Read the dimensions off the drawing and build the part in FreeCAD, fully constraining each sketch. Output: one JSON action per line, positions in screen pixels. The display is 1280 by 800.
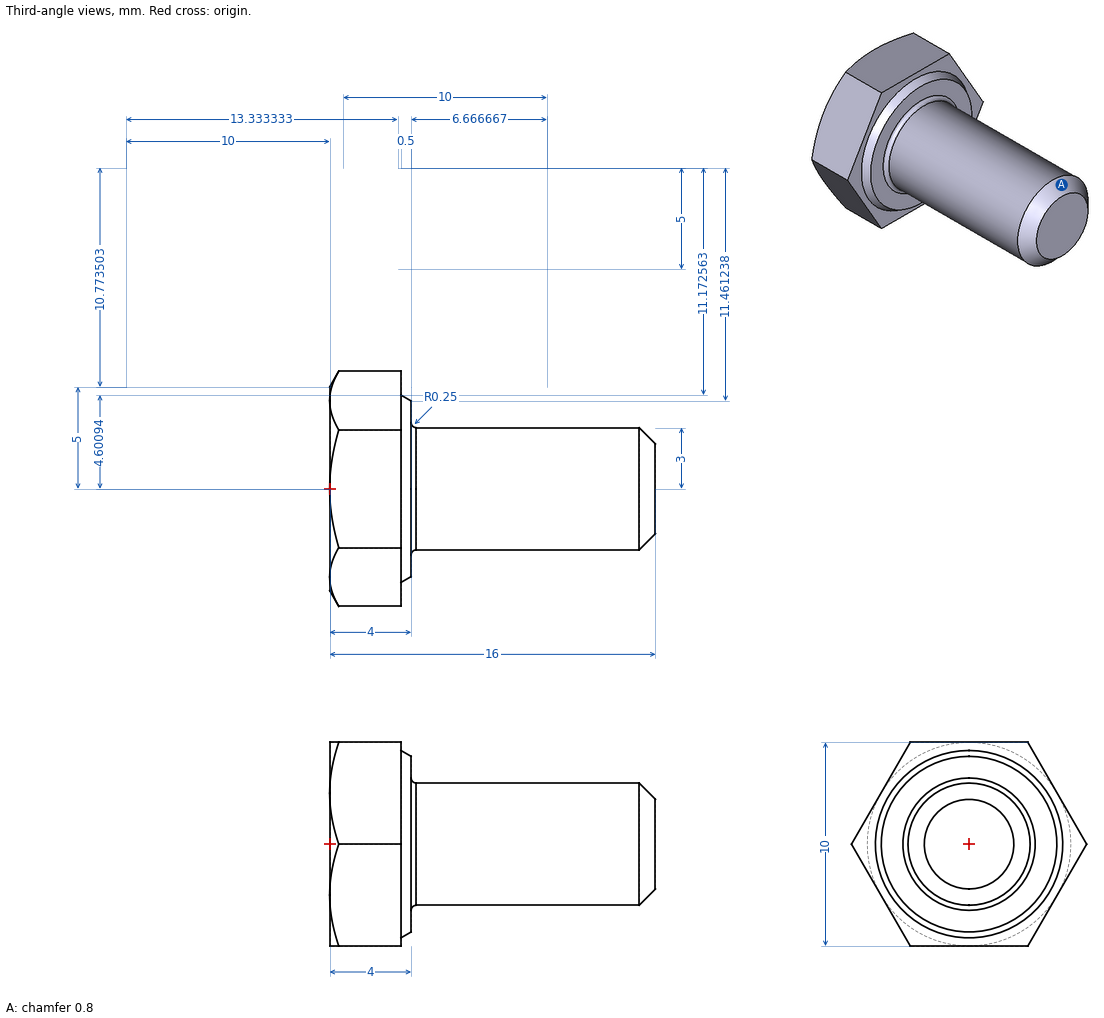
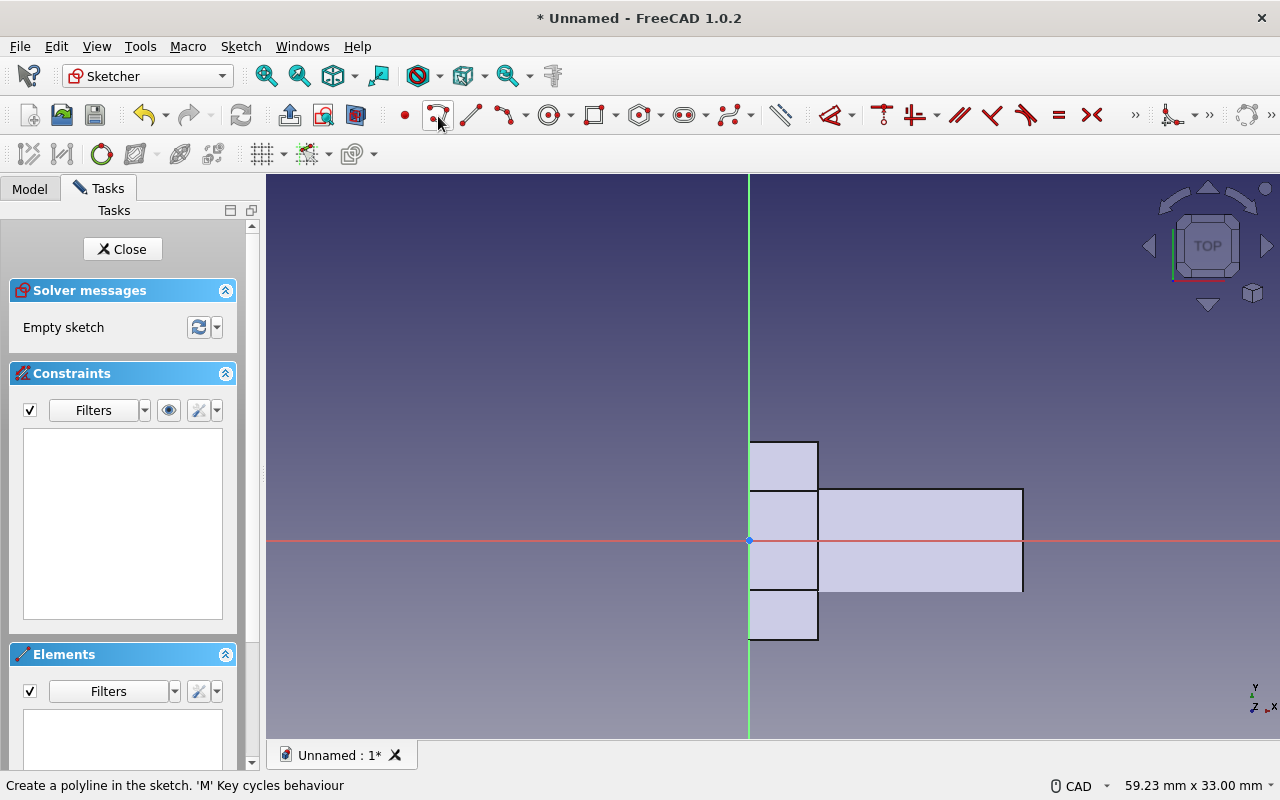
{"action": "left_click", "coordinate": [749, 455]}
{"action": "left_click", "coordinate": [806, 356]}
{"action": "left_click", "coordinate": [806, 271]}
{"action": "left_click", "coordinate": [578, 271]}
{"action": "left_click", "coordinate": [578, 455]}
{"action": "left_click", "coordinate": [749, 456]}
{"action": "key", "text": "Escape"}
{"action": "key", "text": "Escape"}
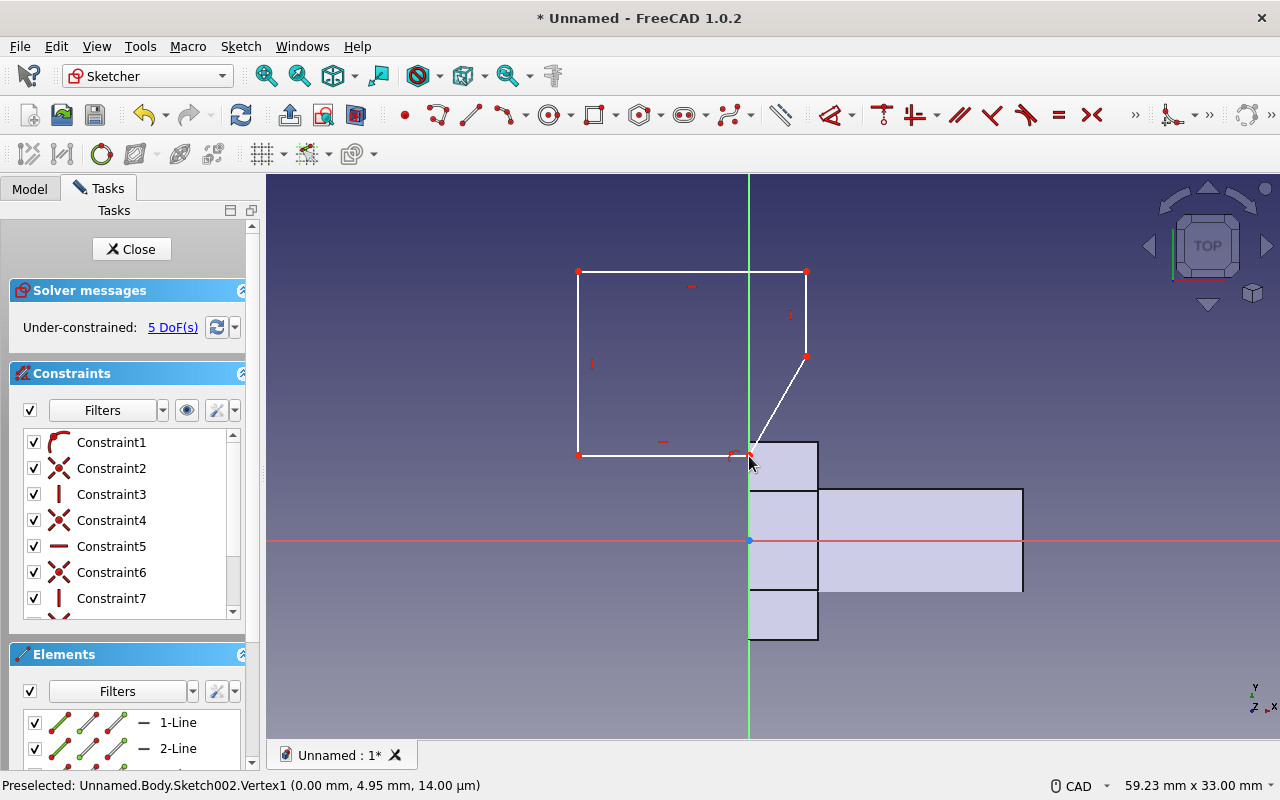
{"action": "left_click", "coordinate": [806, 331]}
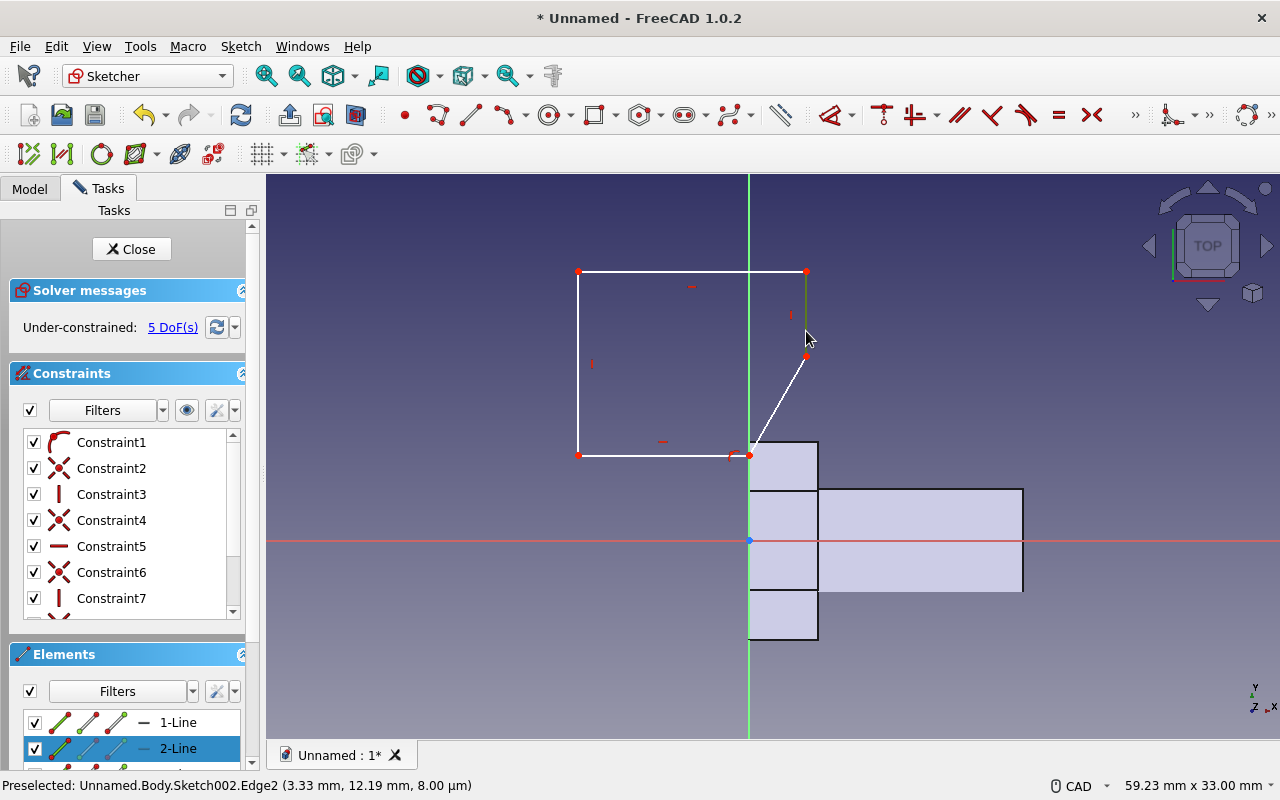
{"action": "key", "text": "i"}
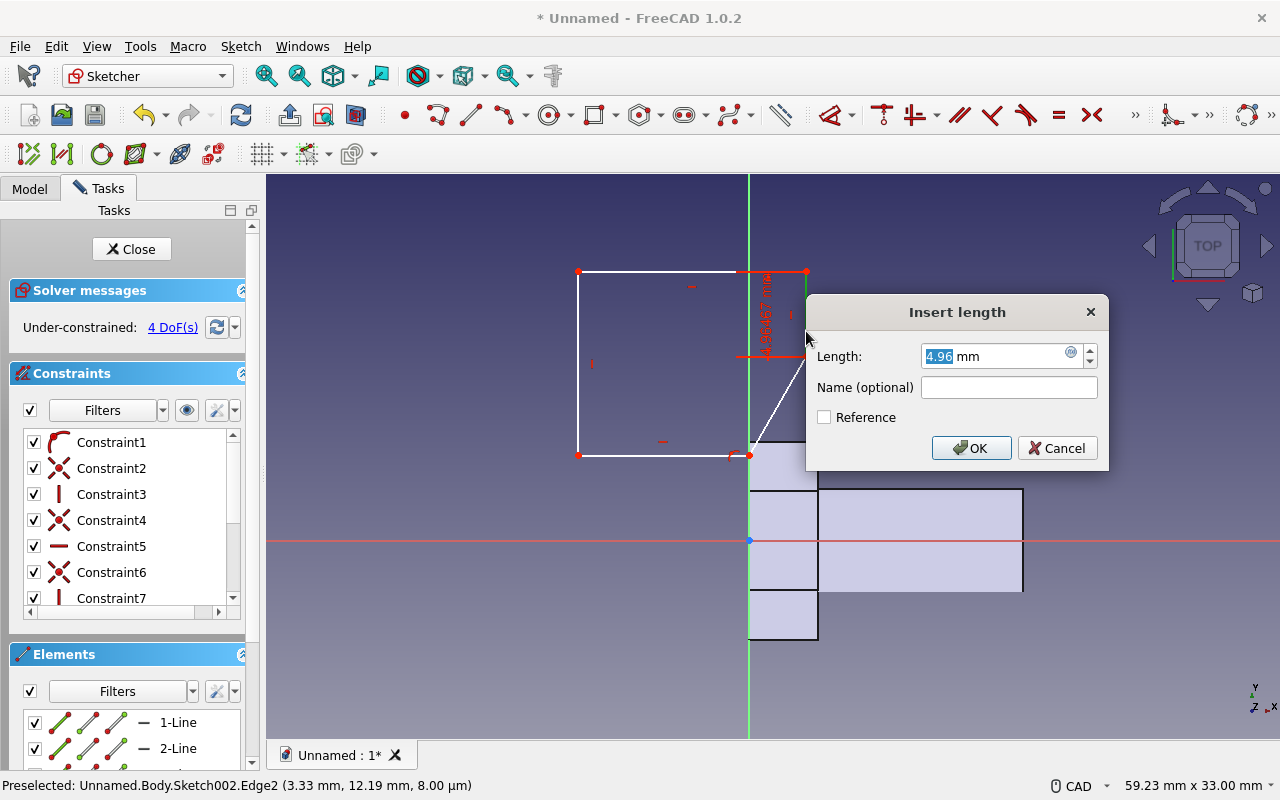
{"action": "type", "text": "5"}
{"action": "key", "text": "Return"}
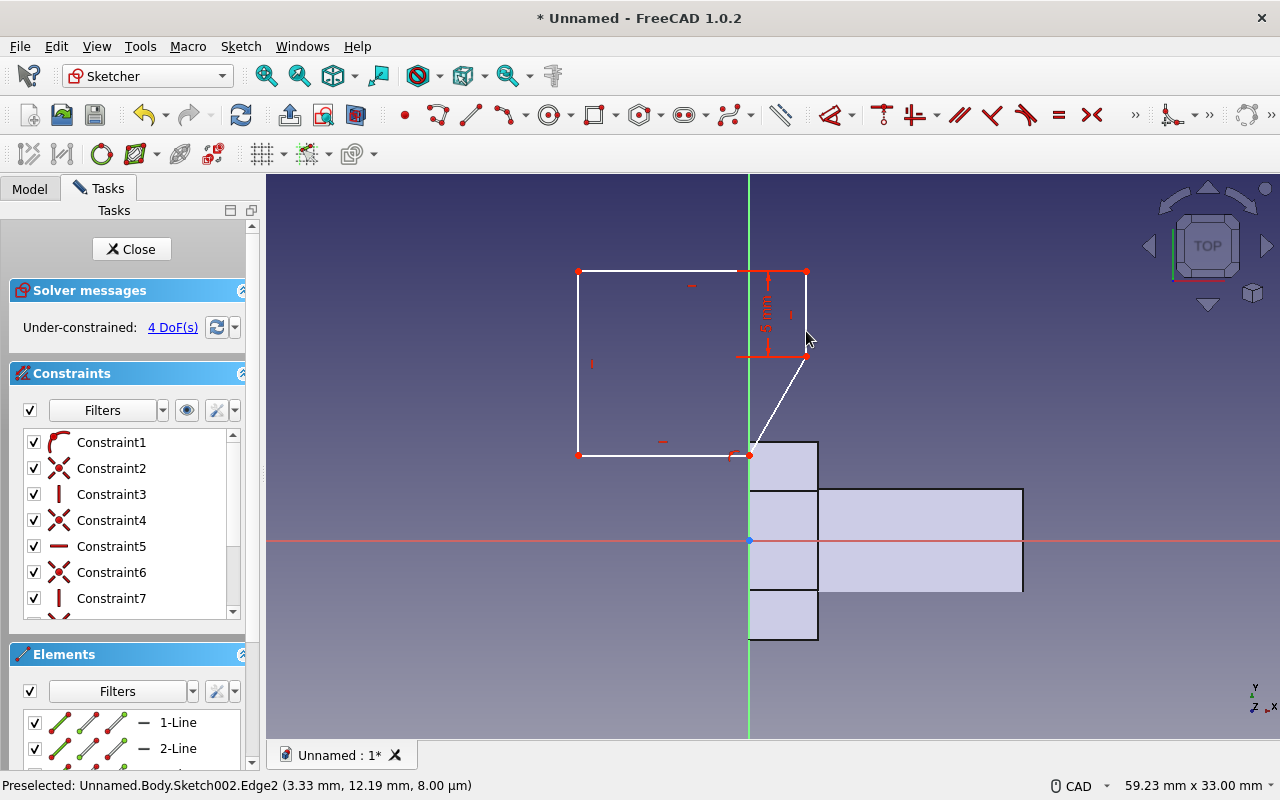
{"action": "left_click", "coordinate": [629, 456]}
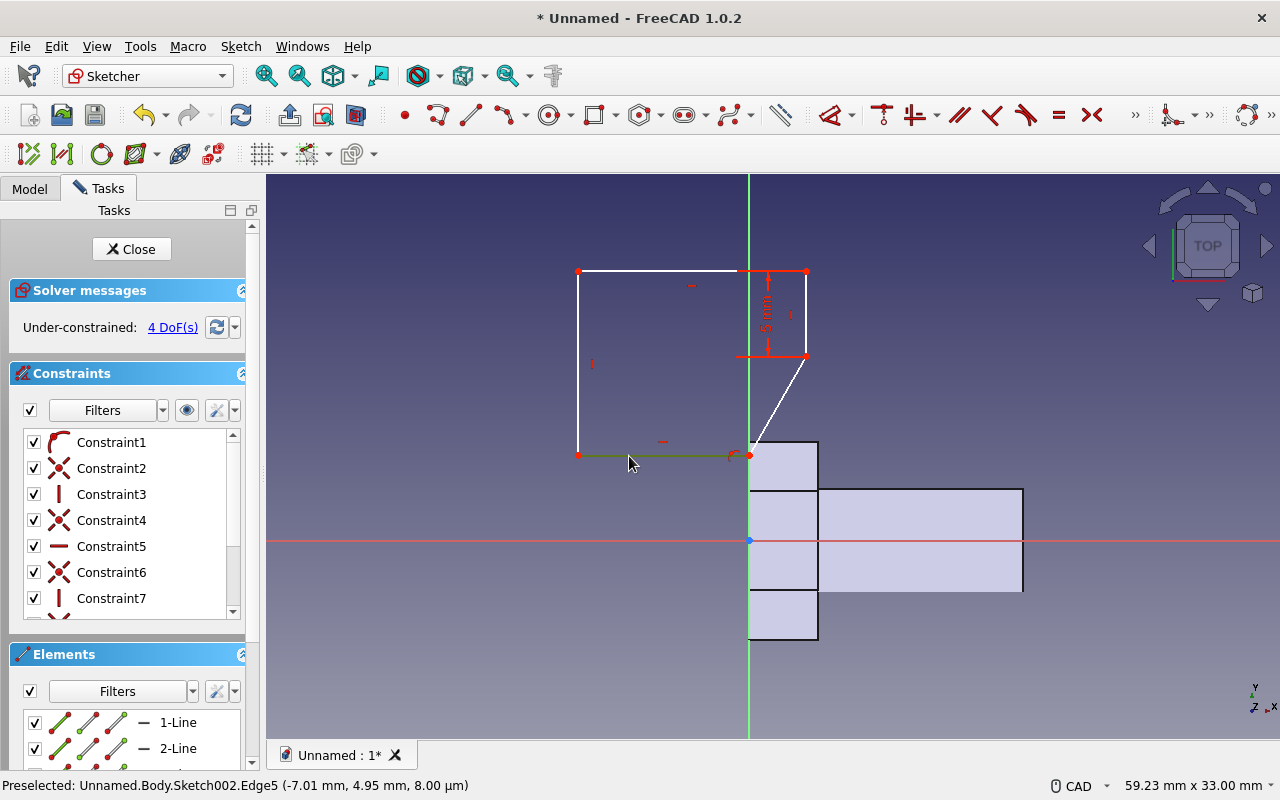
{"action": "left_click", "coordinate": [852, 116]}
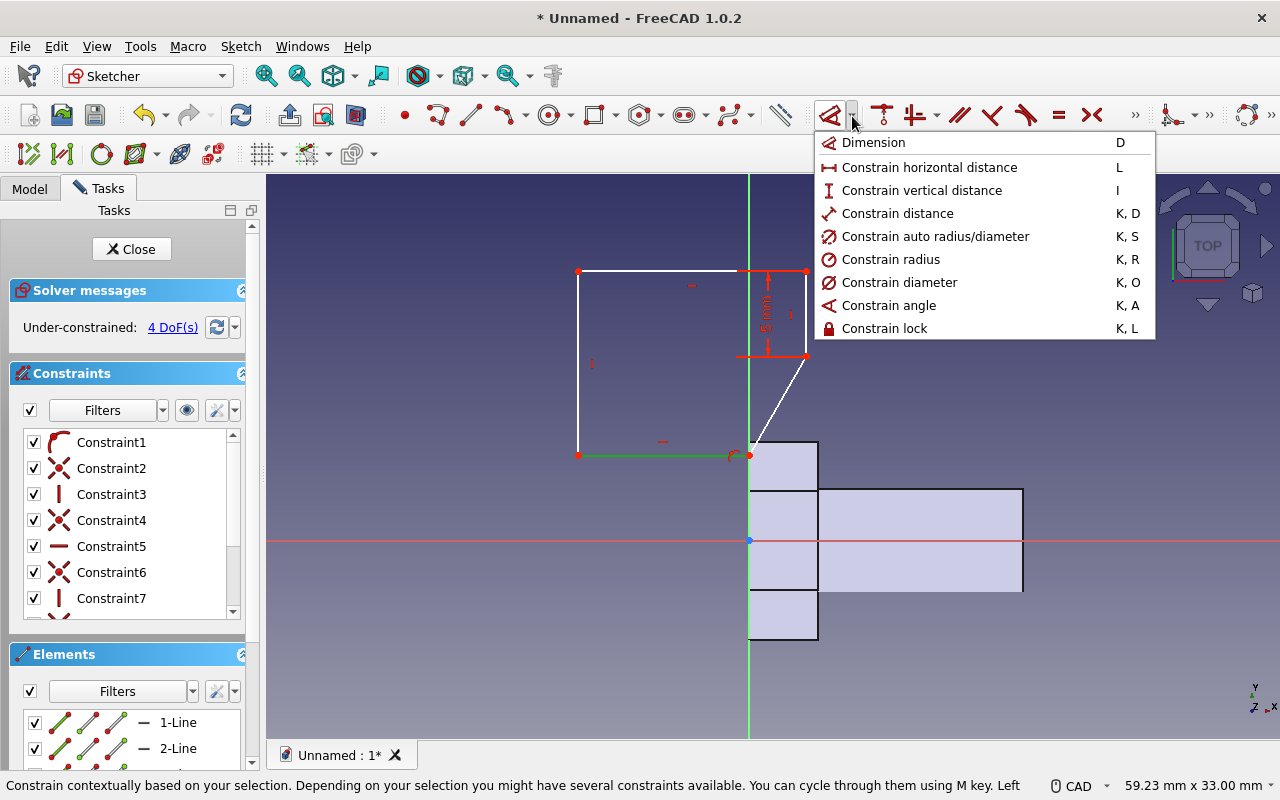
{"action": "left_click", "coordinate": [985, 168]}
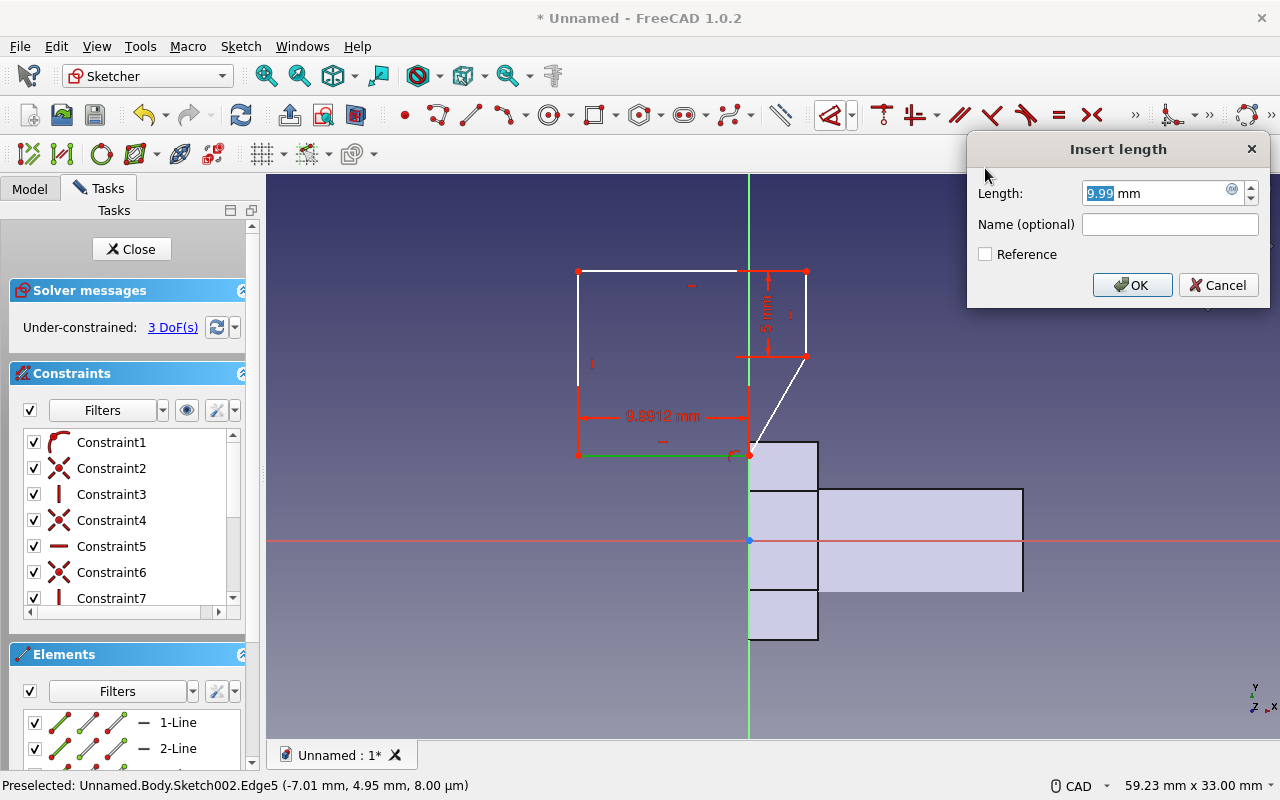
{"action": "type", "text": "10"}
{"action": "key", "text": "Return"}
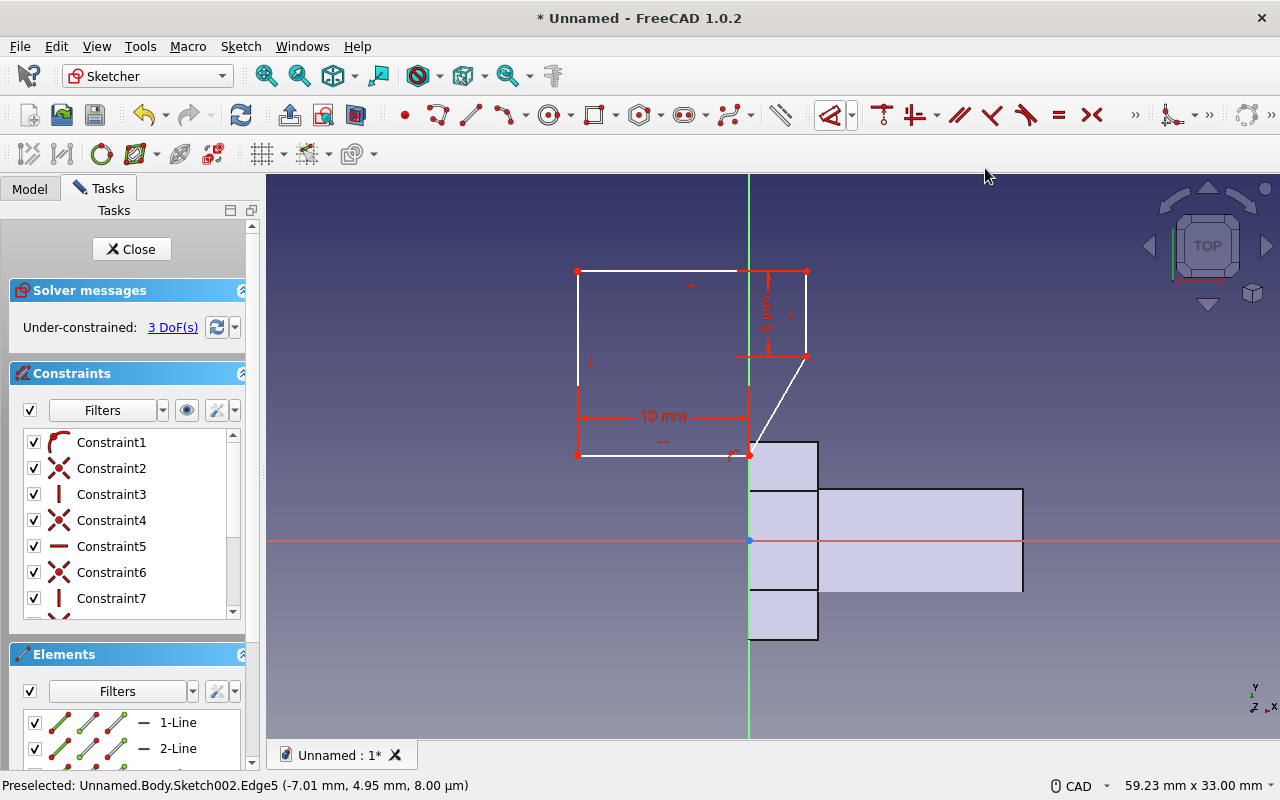
{"action": "left_click", "coordinate": [749, 456]}